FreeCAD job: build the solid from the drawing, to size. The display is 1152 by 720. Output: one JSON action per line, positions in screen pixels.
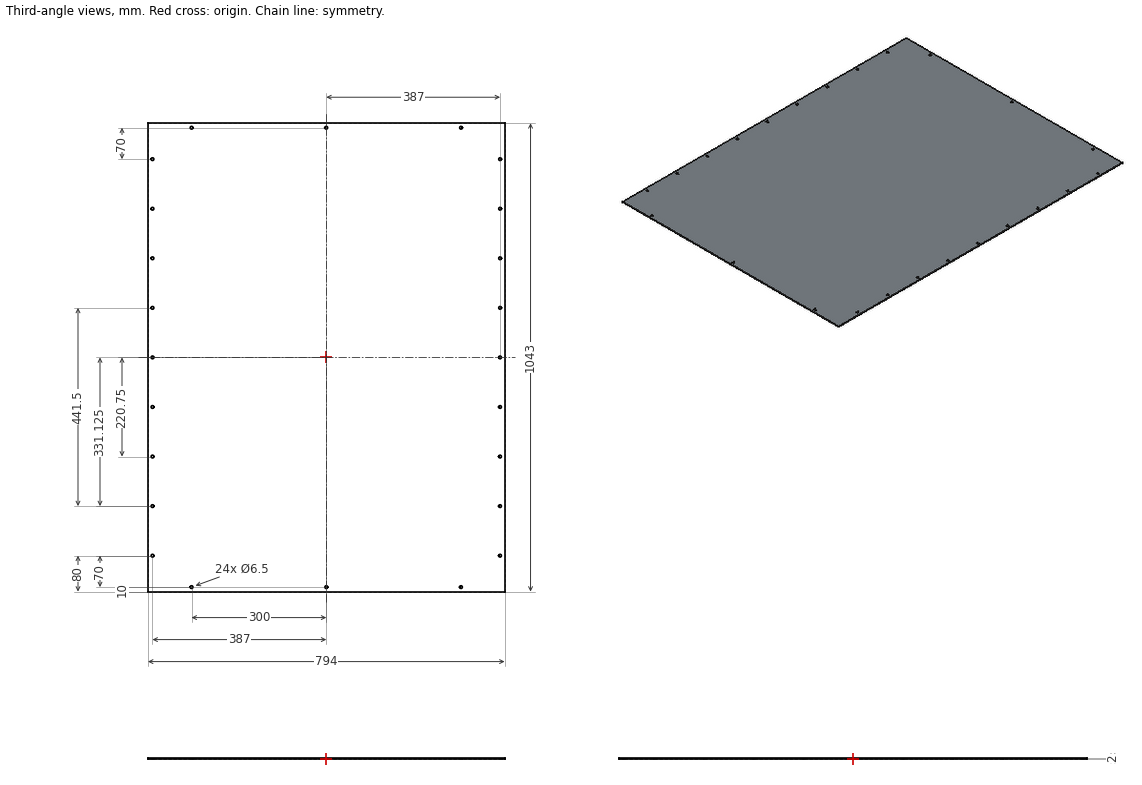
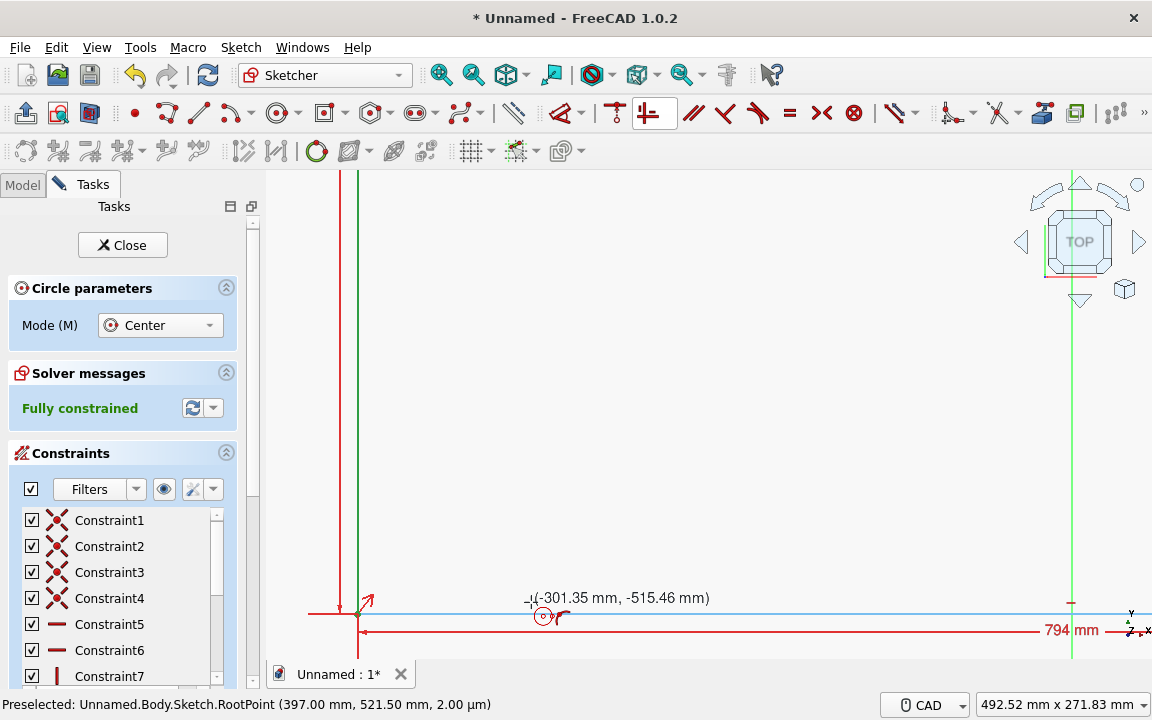
{"action": "left_click", "coordinate": [532, 596]}
{"action": "mouse_move", "coordinate": [536, 592]}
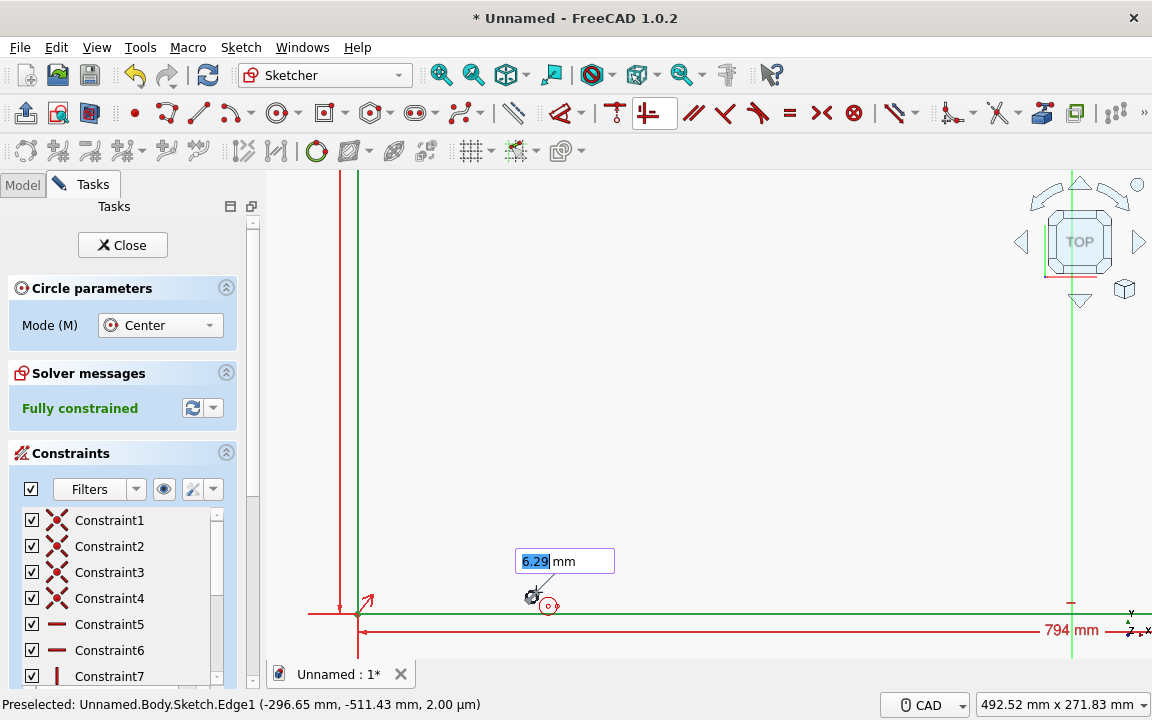
{"action": "type", "text": "6.5"}
{"action": "key", "text": "Return"}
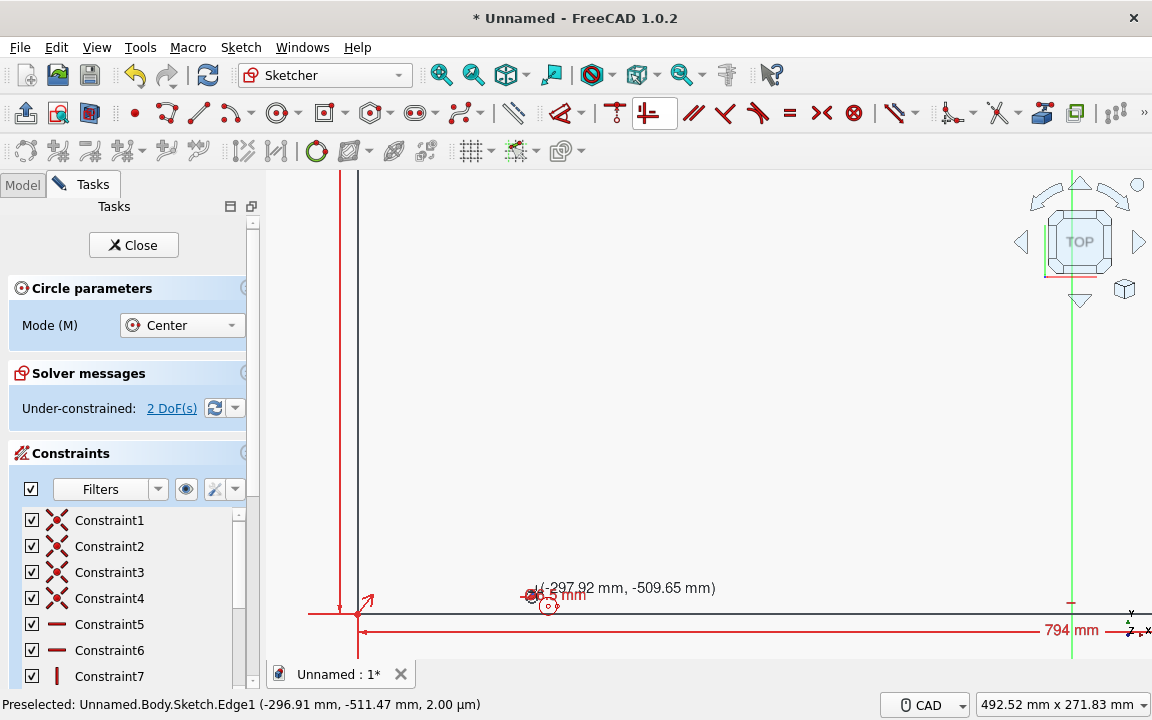
{"action": "scroll", "coordinate": [376, 470], "scroll_direction": "up", "scroll_amount": 7}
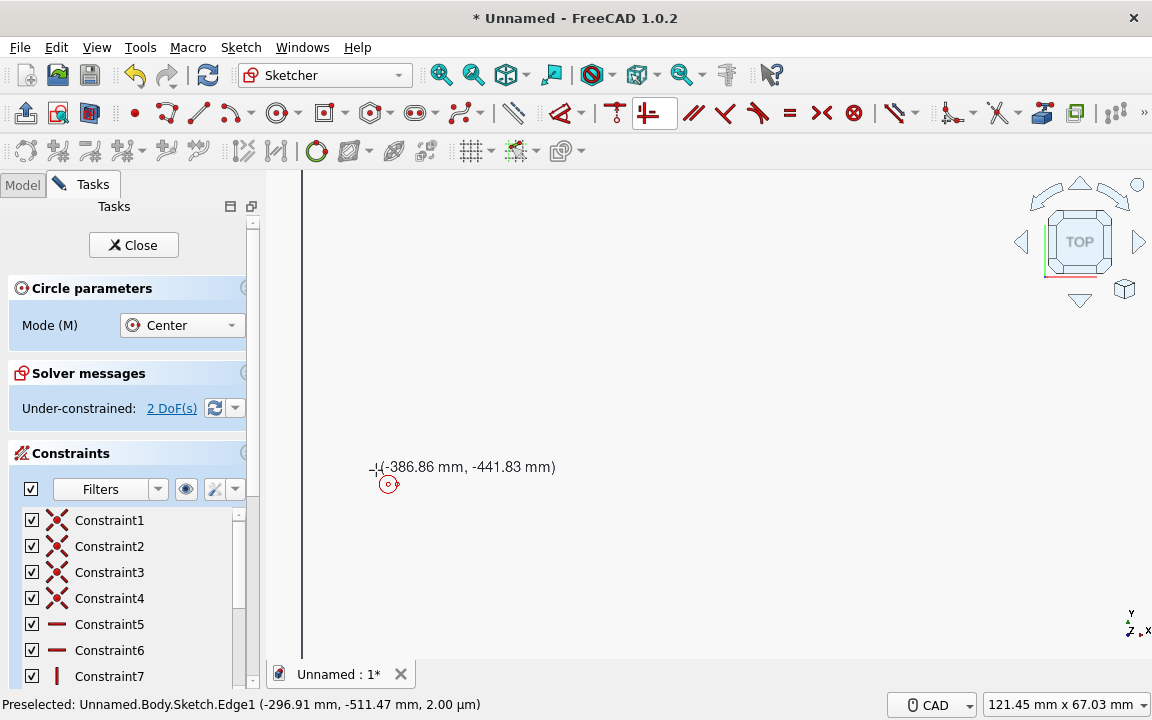
{"action": "scroll", "coordinate": [507, 580], "scroll_direction": "down", "scroll_amount": 15}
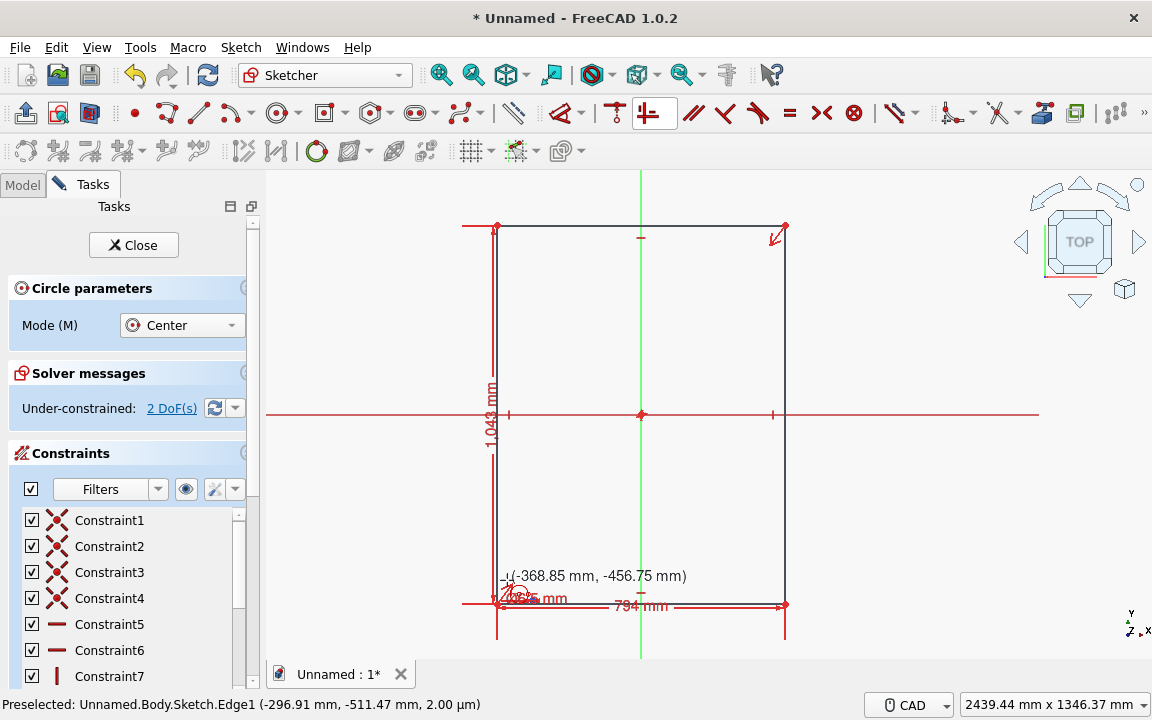
{"action": "scroll", "coordinate": [501, 575], "scroll_direction": "up", "scroll_amount": 8}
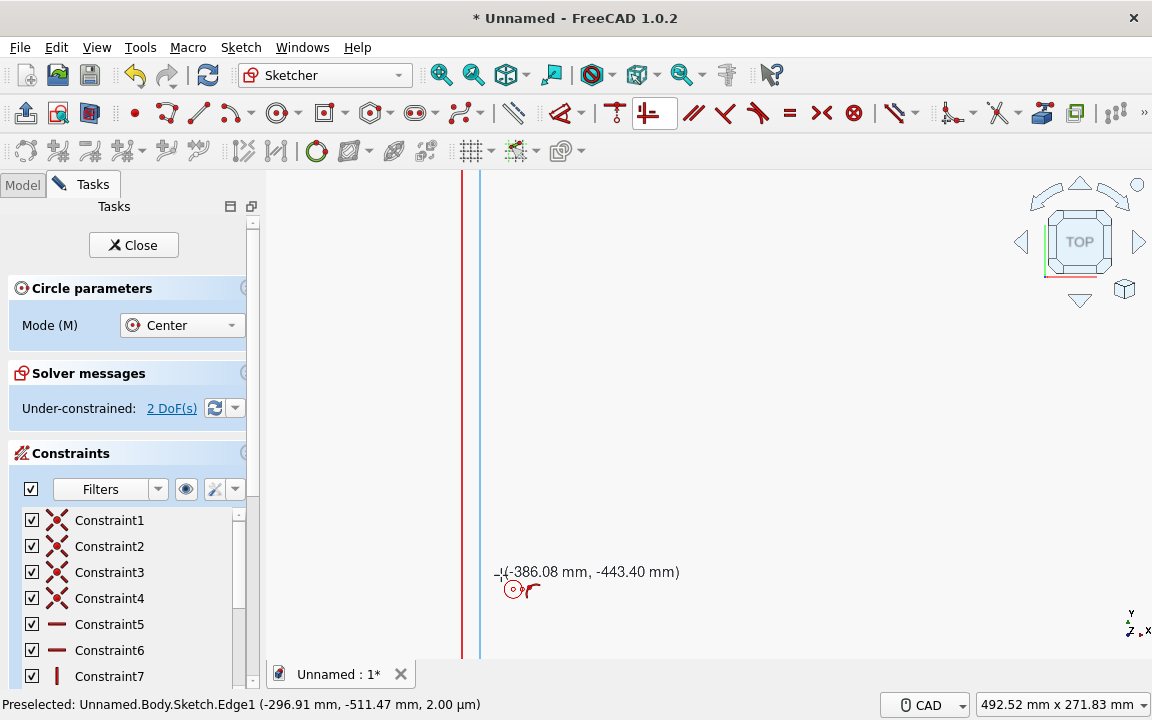
{"action": "left_click", "coordinate": [498, 573]}
{"action": "mouse_move", "coordinate": [502, 569]}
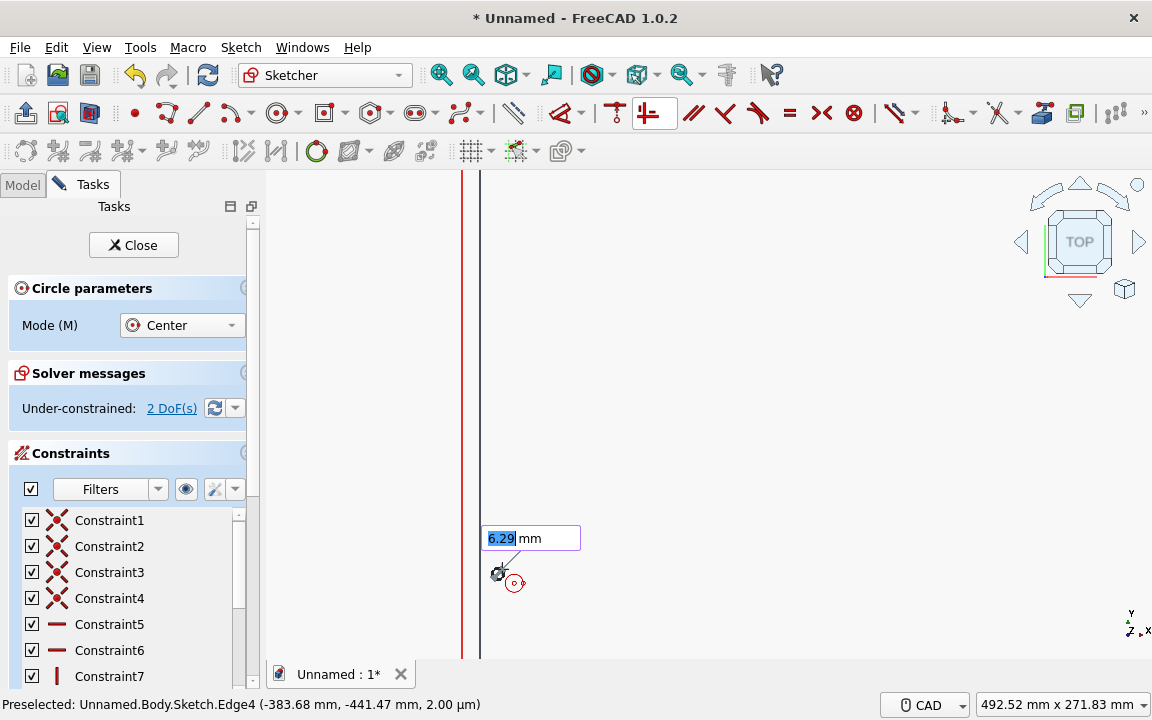
{"action": "type", "text": "6.5"}
{"action": "key", "text": "Return"}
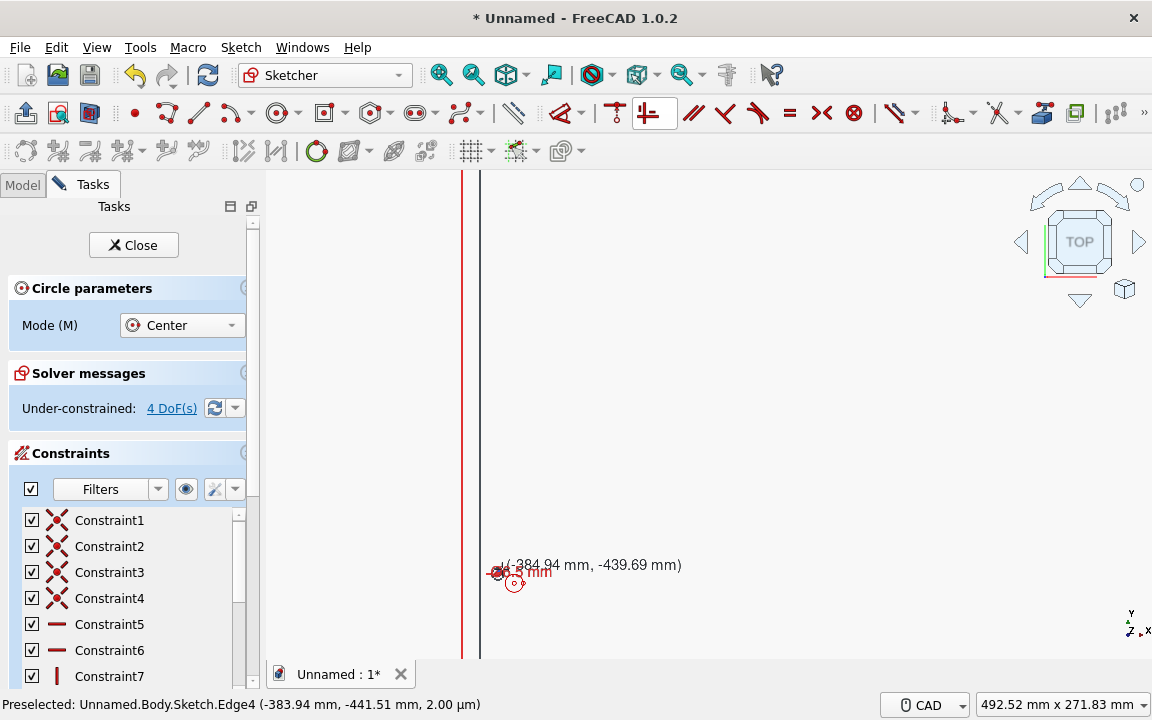
{"action": "scroll", "coordinate": [498, 375], "scroll_direction": "up", "scroll_amount": 7}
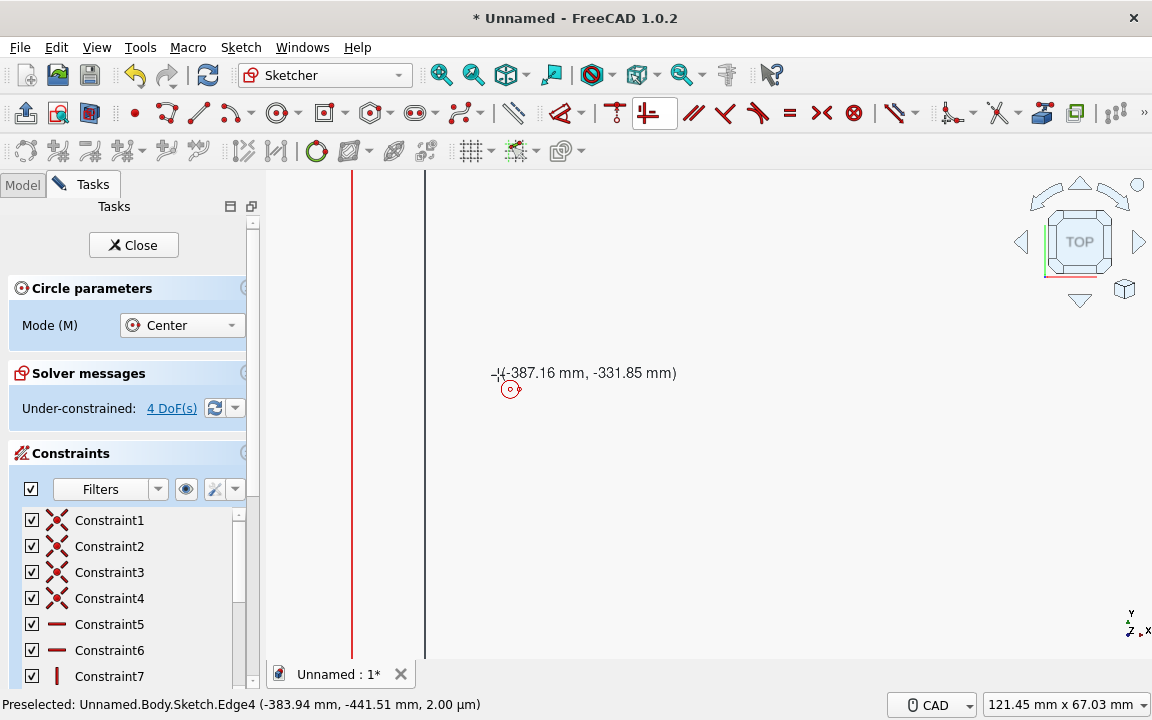
{"action": "scroll", "coordinate": [500, 543], "scroll_direction": "down", "scroll_amount": 15}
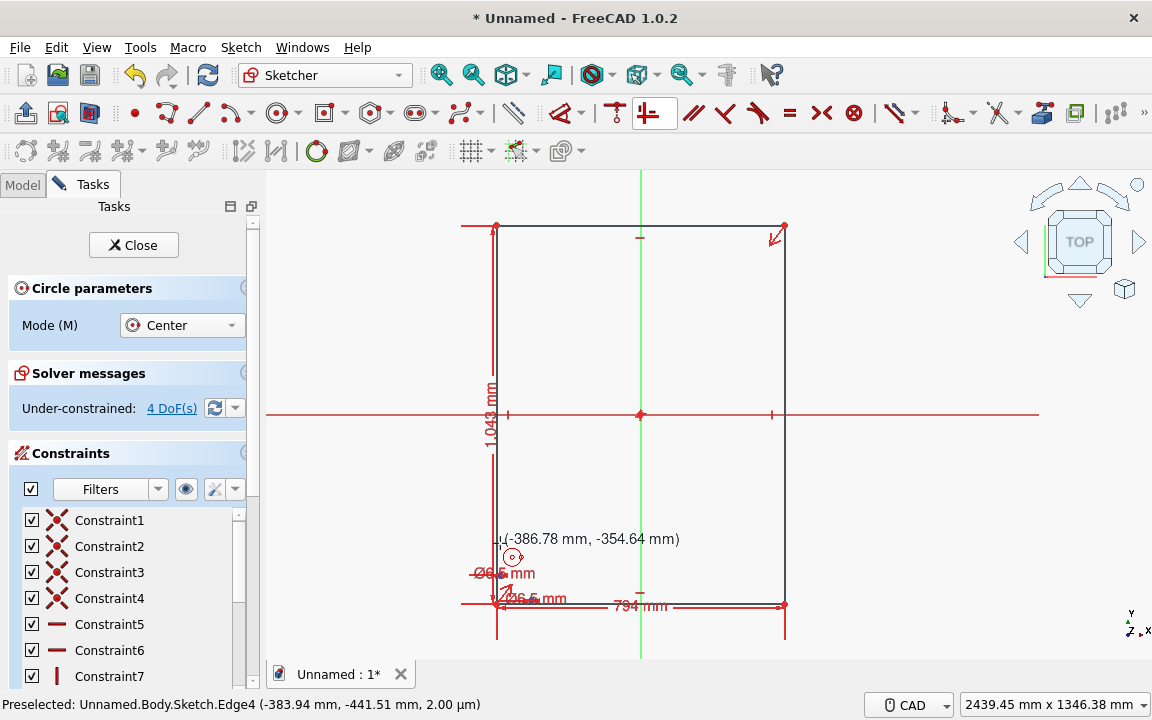
{"action": "scroll", "coordinate": [500, 535], "scroll_direction": "up", "scroll_amount": 8}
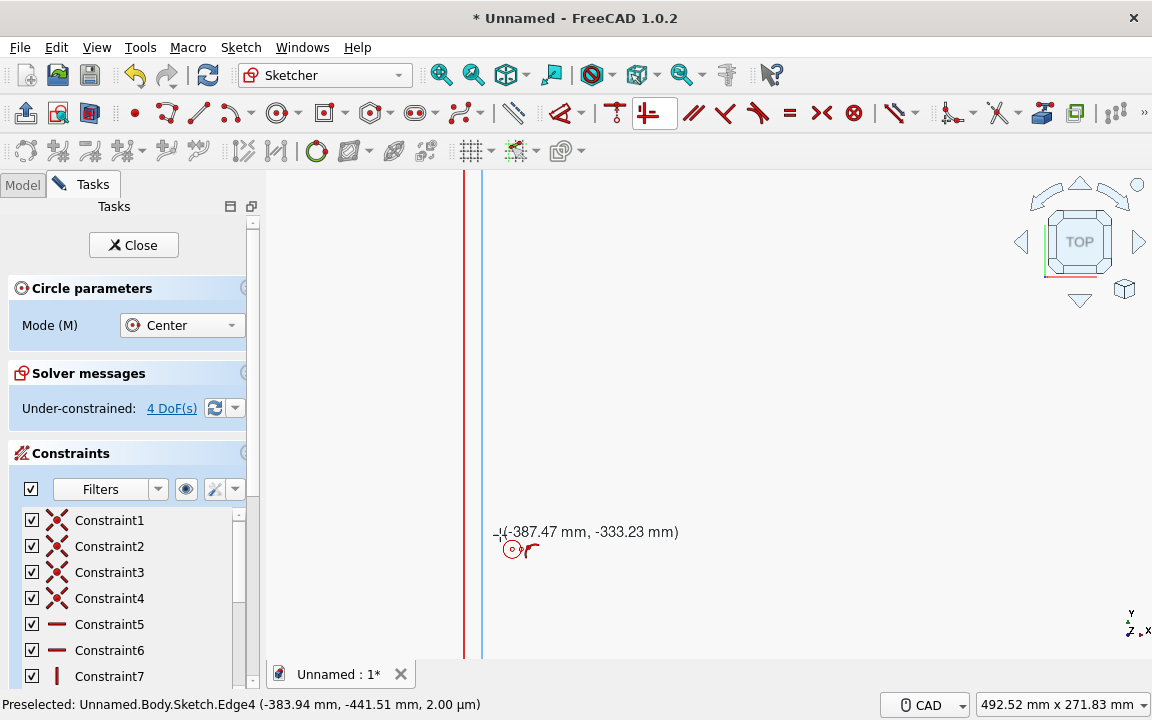
{"action": "left_click", "coordinate": [500, 533]}
{"action": "mouse_move", "coordinate": [504, 529]}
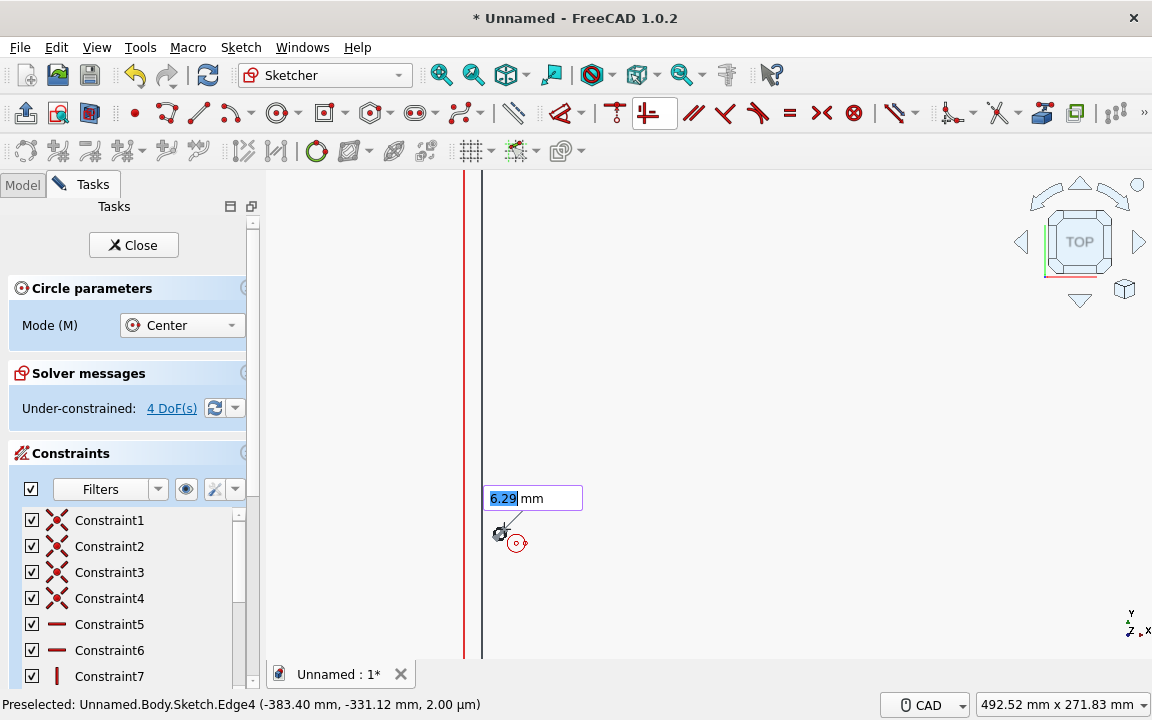
{"action": "type", "text": "6.5"}
{"action": "key", "text": "Return"}